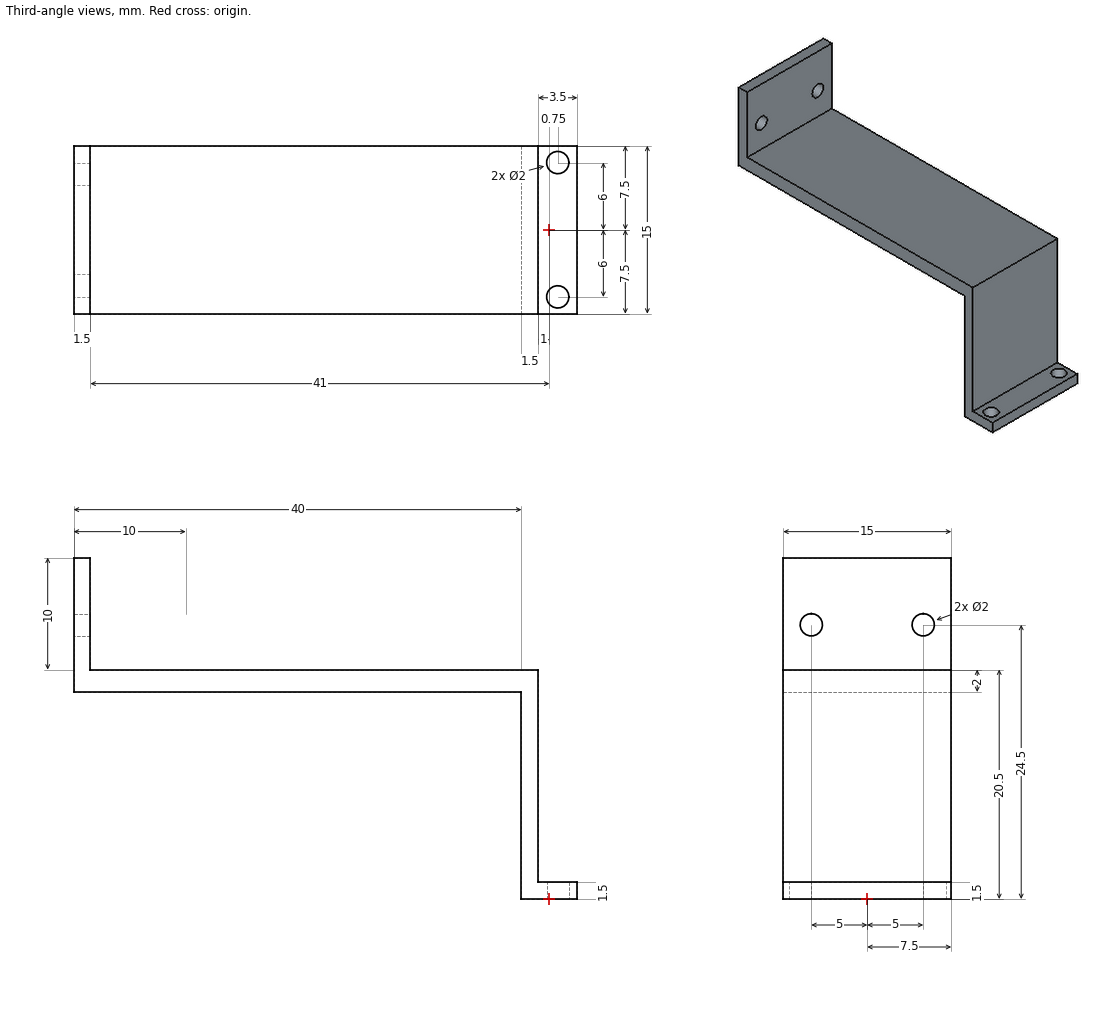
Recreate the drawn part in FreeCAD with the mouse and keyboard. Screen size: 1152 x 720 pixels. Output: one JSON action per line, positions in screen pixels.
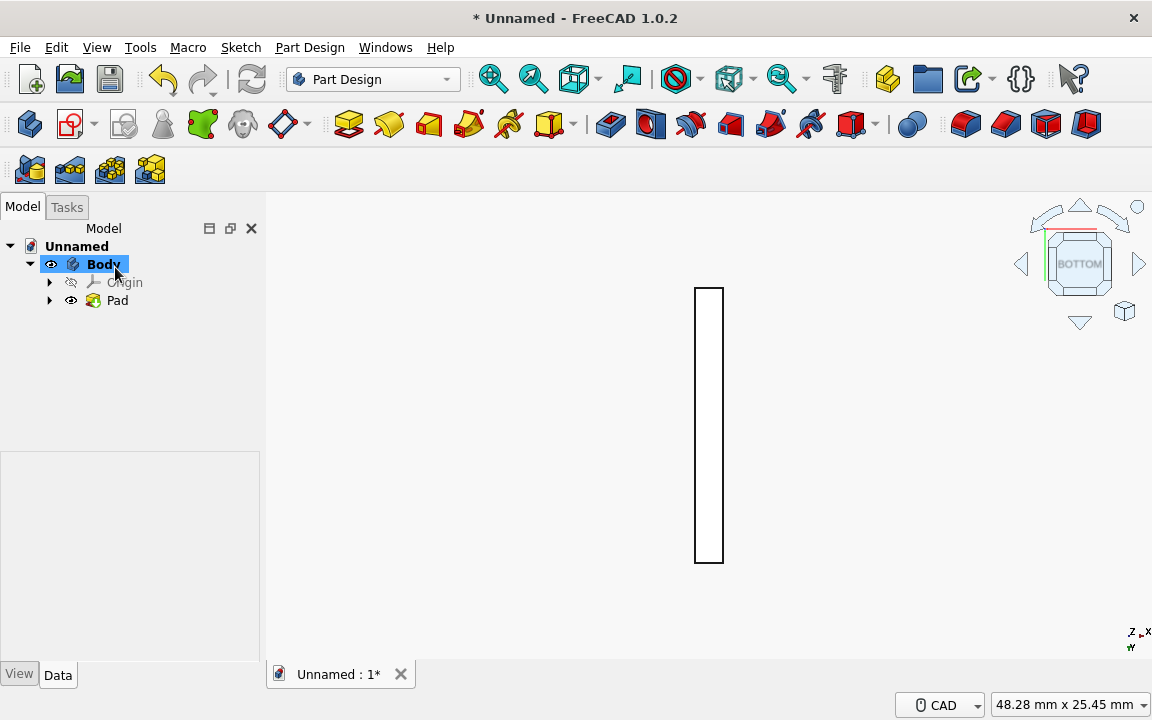
{"action": "left_click", "coordinate": [709, 542]}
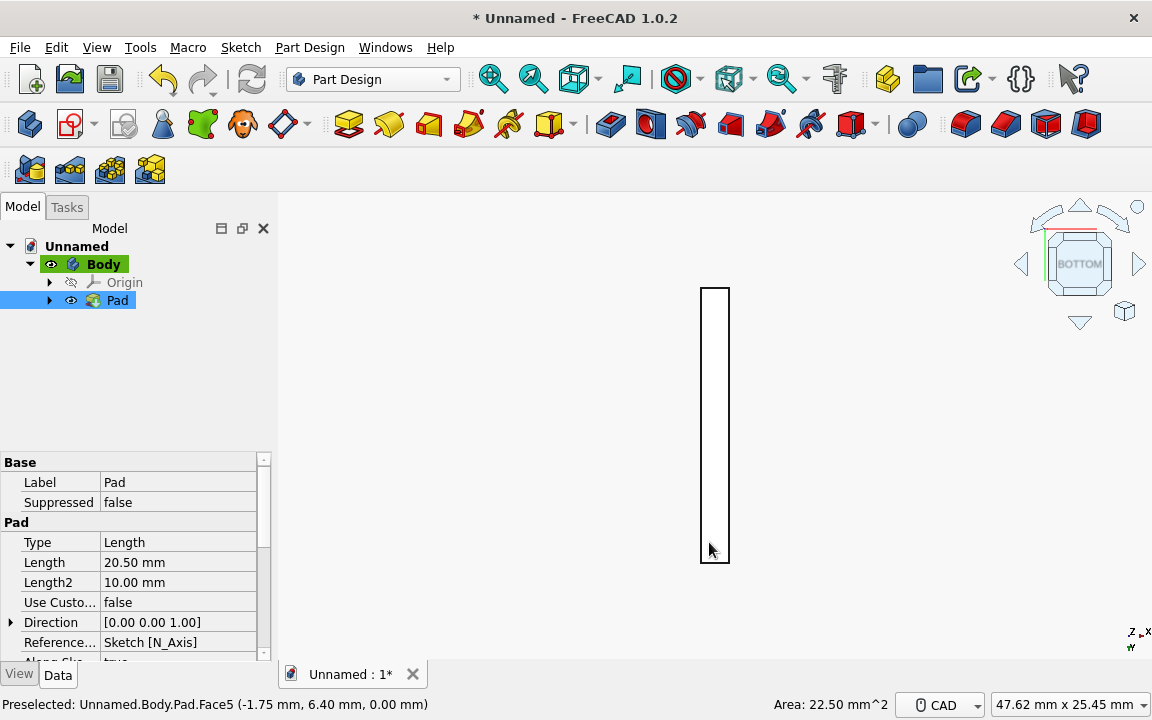
{"action": "left_click", "coordinate": [70, 124]}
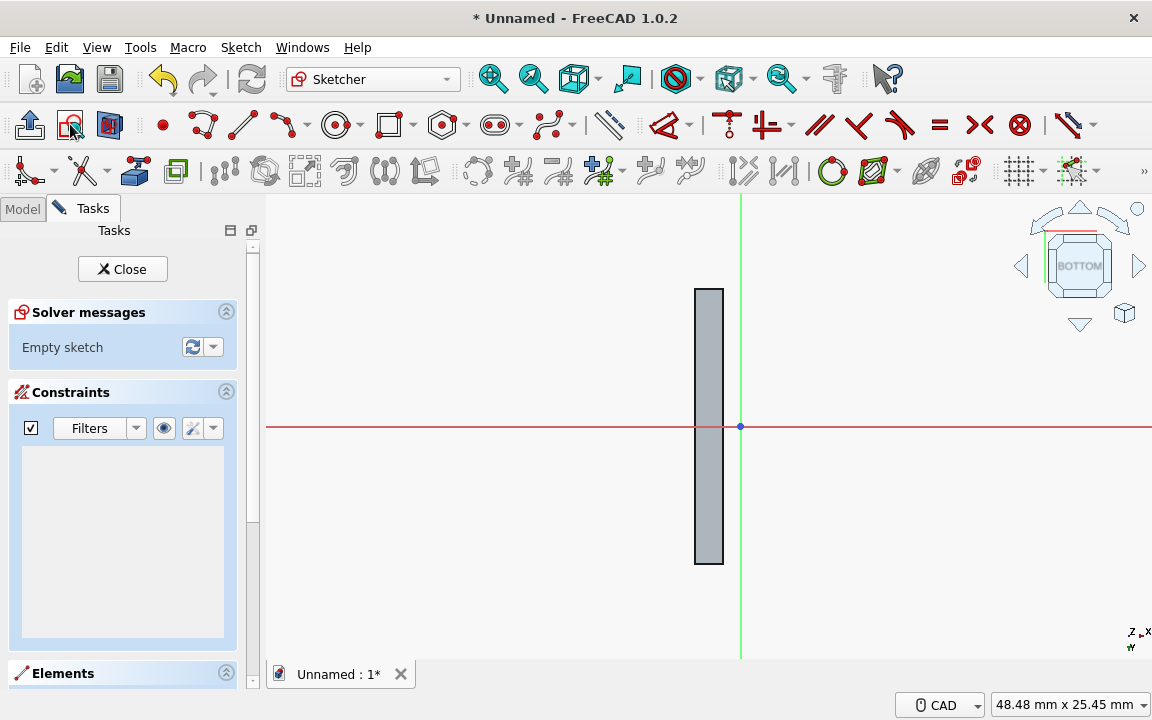
{"action": "left_click", "coordinate": [390, 126]}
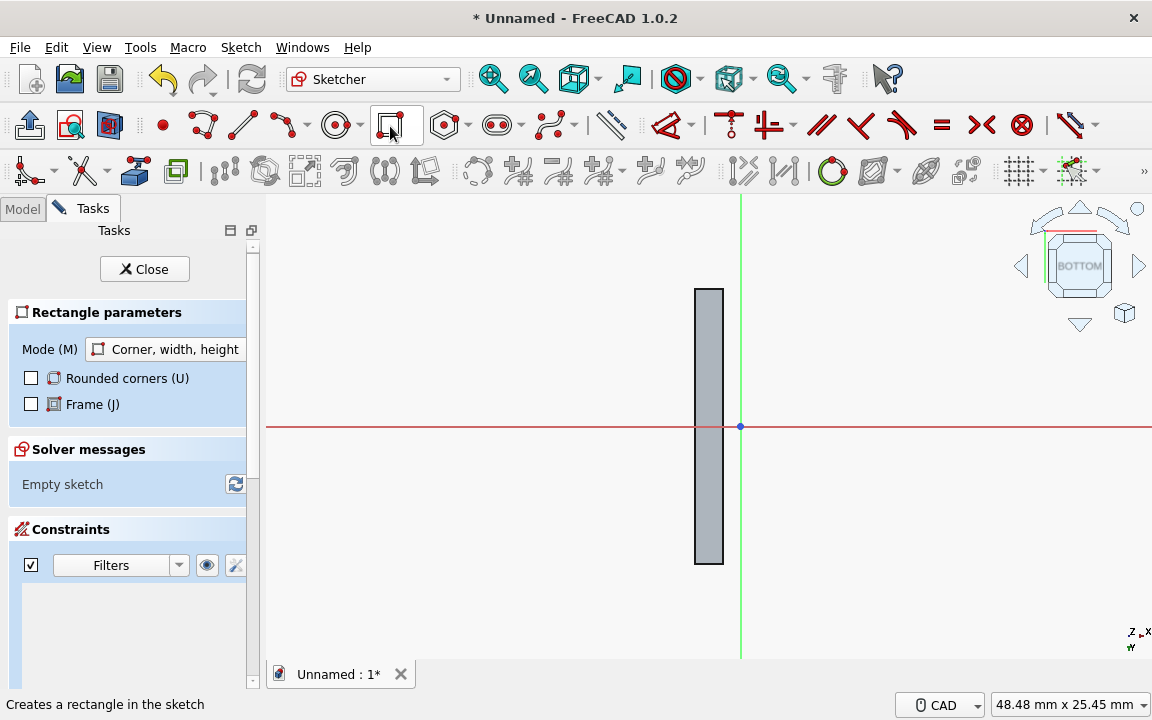
{"action": "left_click", "coordinate": [723, 289]}
{"action": "left_click", "coordinate": [787, 564]}
{"action": "key", "text": "Escape"}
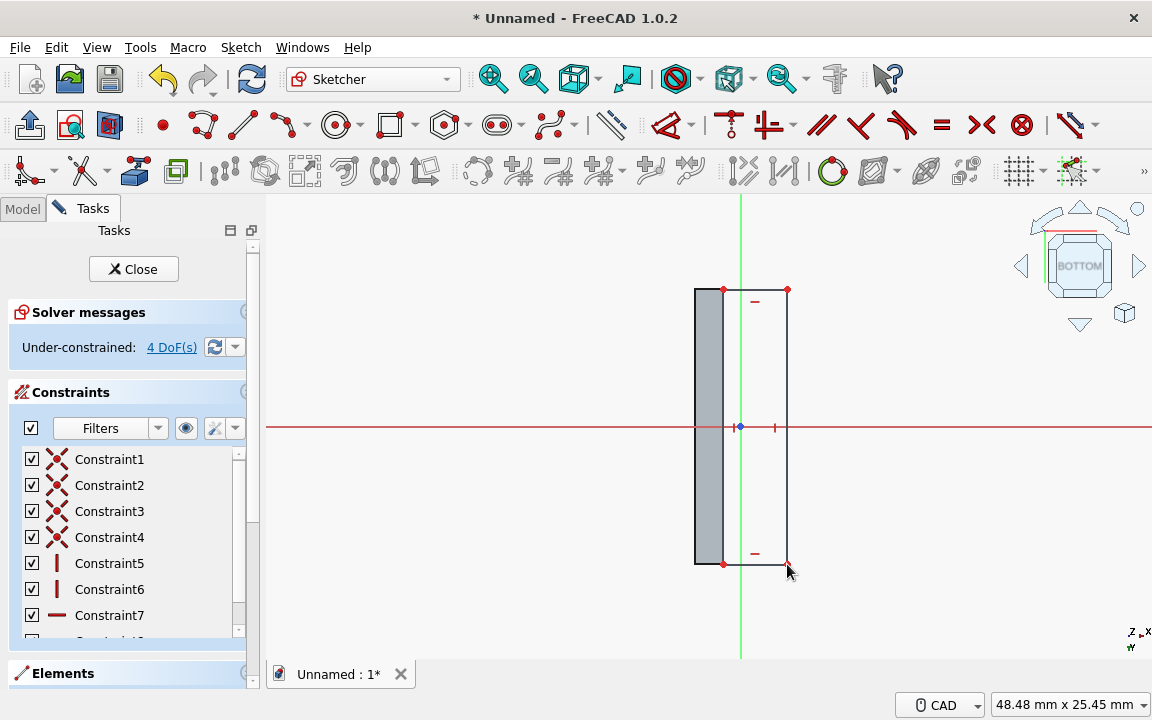
{"action": "left_click", "coordinate": [666, 126]}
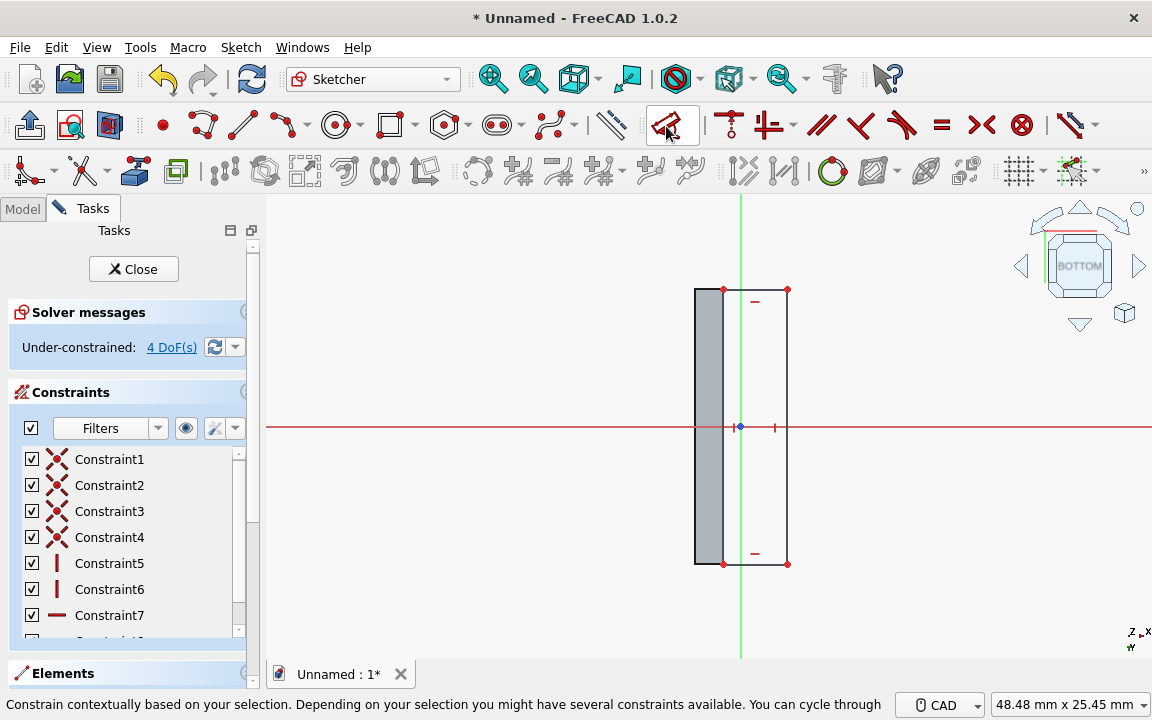
{"action": "left_click", "coordinate": [723, 372]}
{"action": "left_click", "coordinate": [689, 364]}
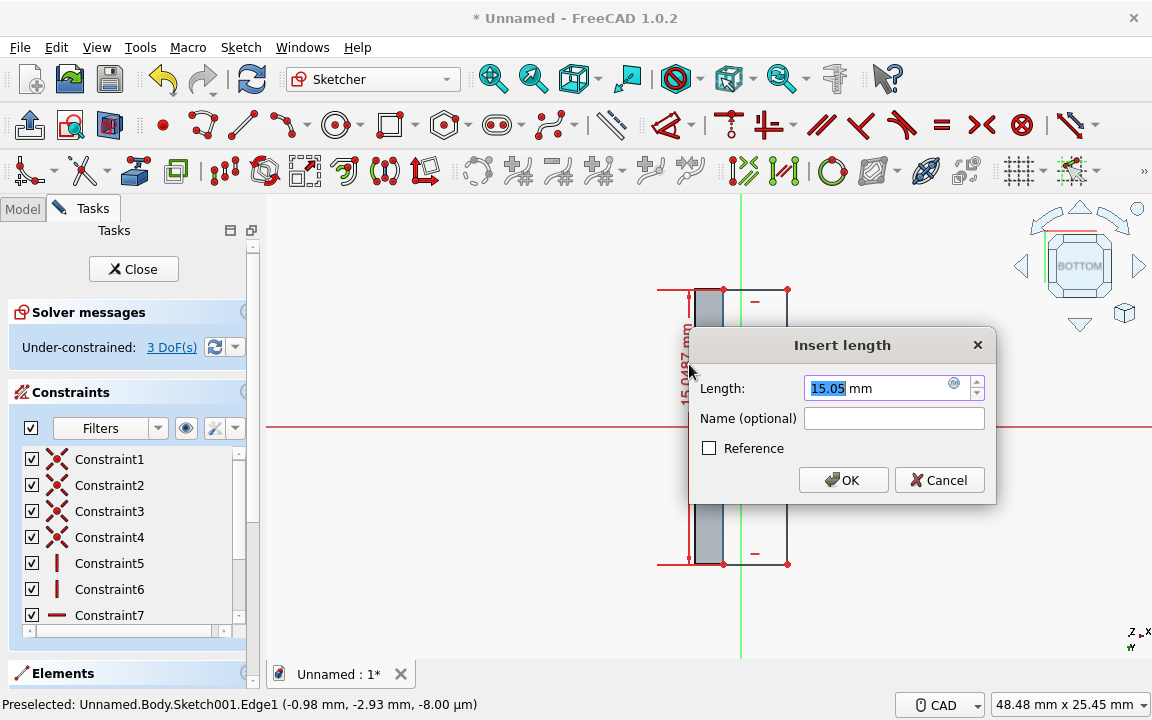
{"action": "type", "text": "15"}
{"action": "key", "text": "Return"}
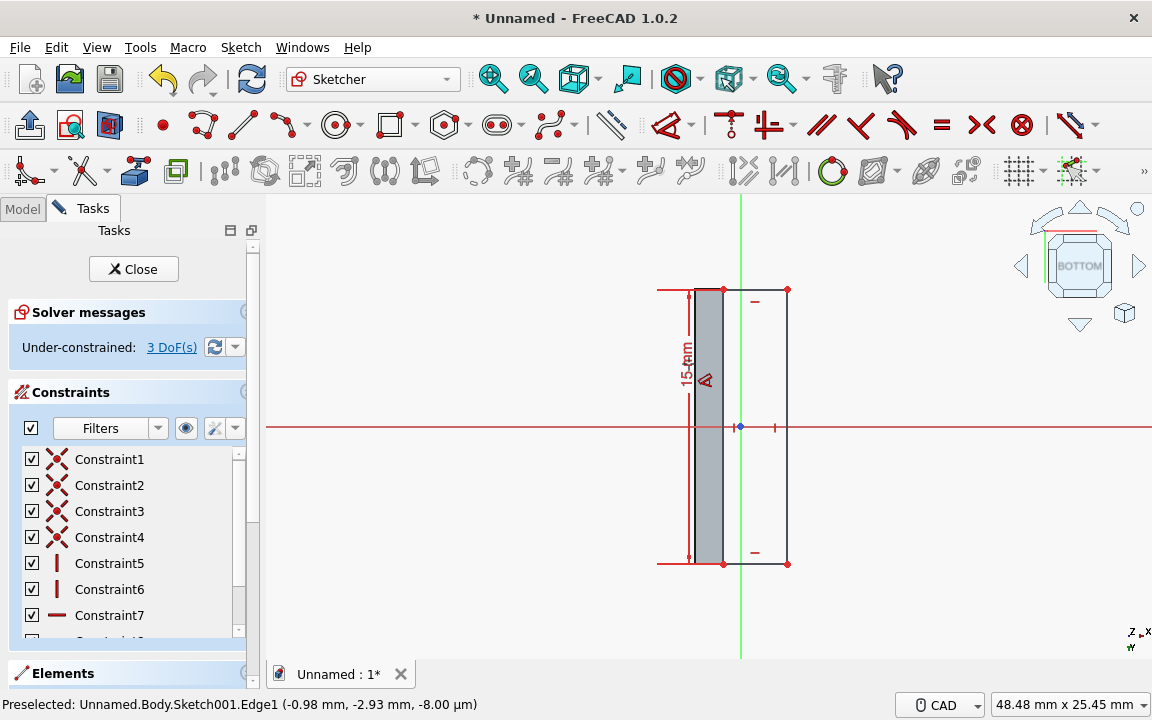
{"action": "scroll", "coordinate": [723, 290], "scroll_direction": "up", "scroll_amount": 4}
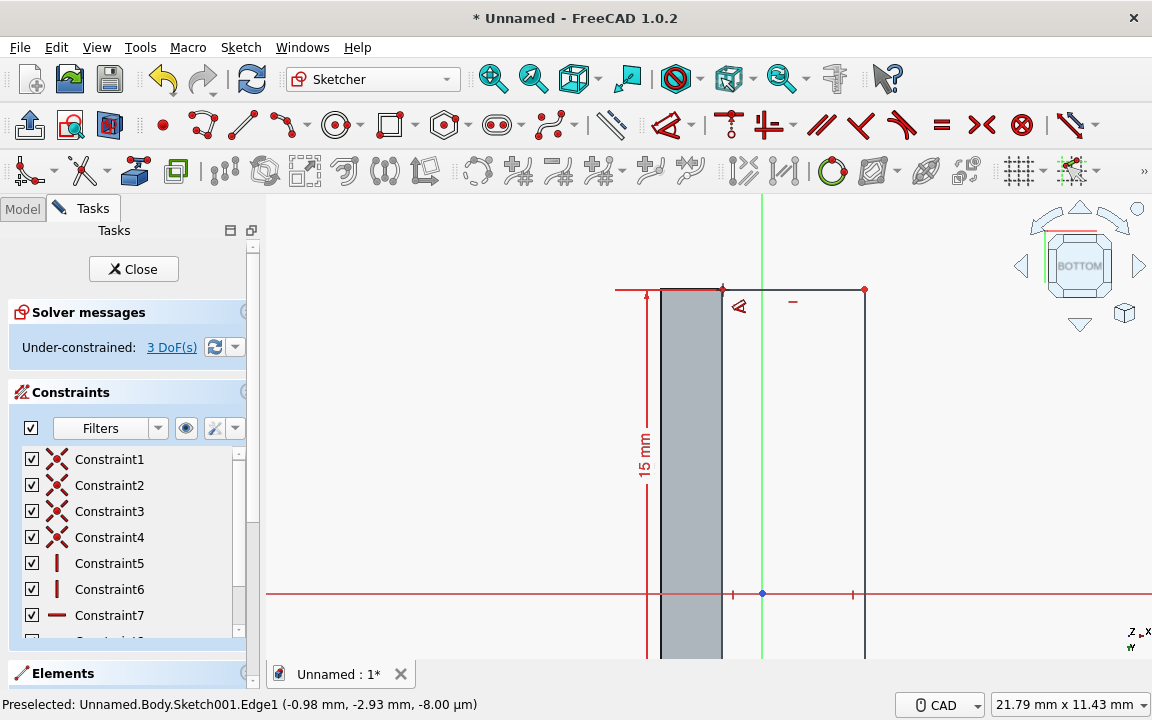
{"action": "left_click", "coordinate": [722, 290]}
{"action": "left_click", "coordinate": [742, 256]}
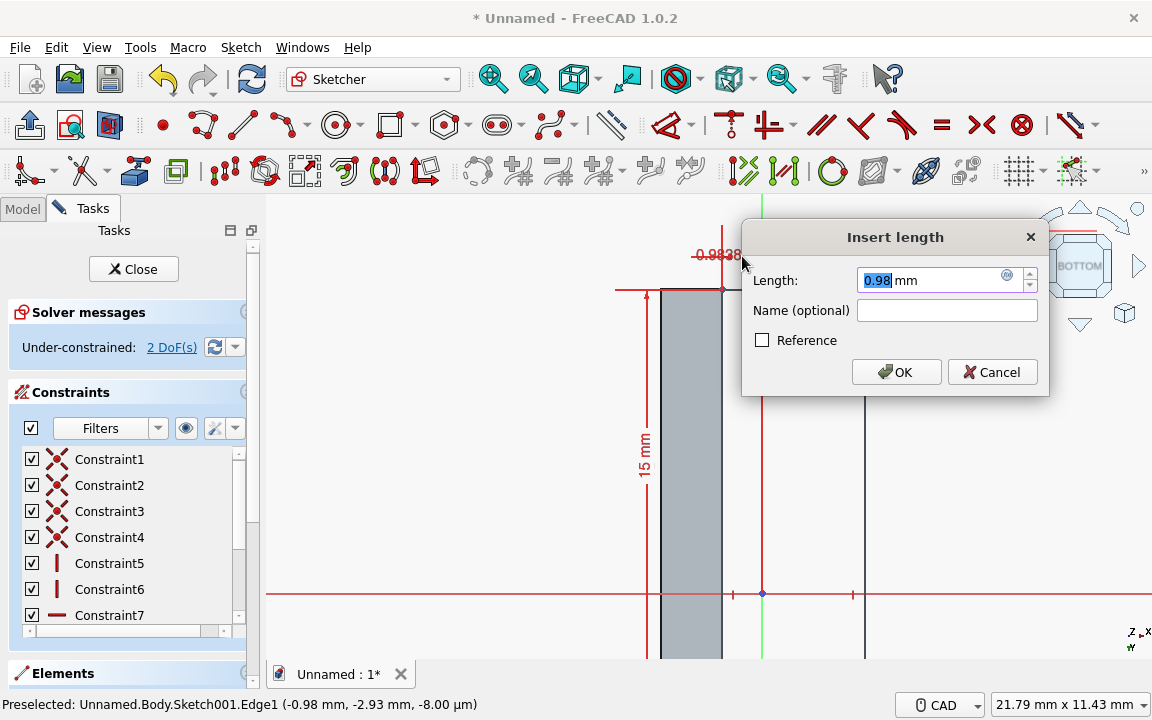
{"action": "type", "text": "1"}
{"action": "key", "text": "Return"}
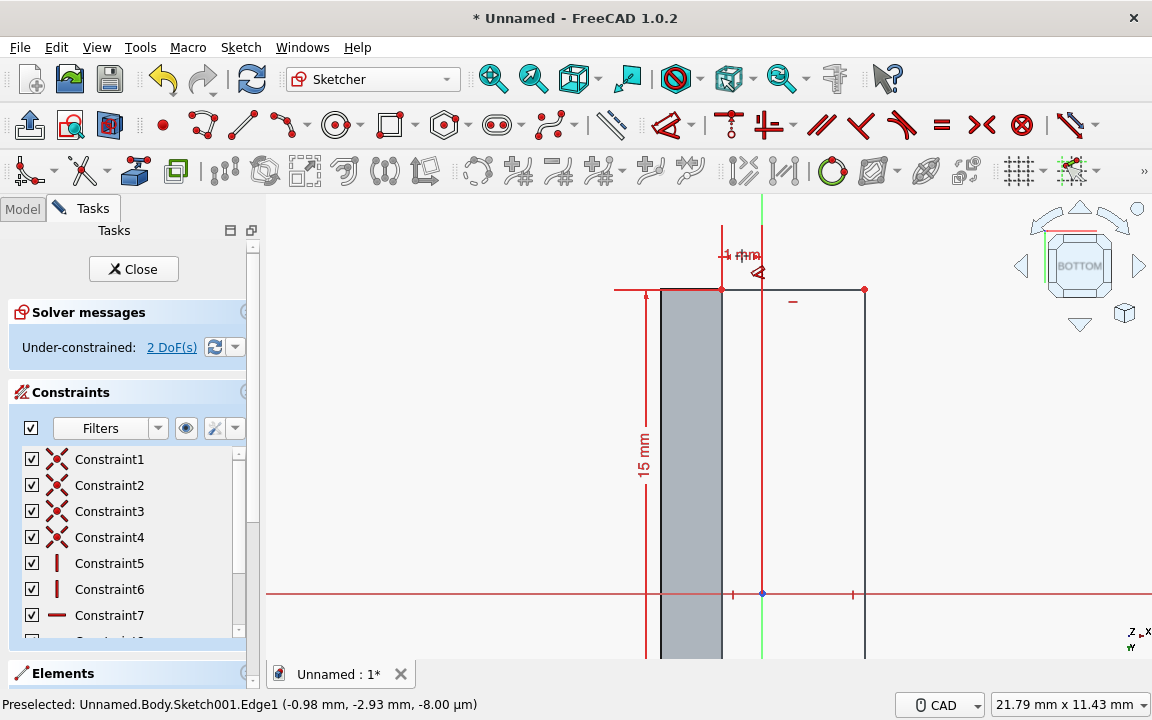
{"action": "scroll", "coordinate": [516, 290], "scroll_direction": "down", "scroll_amount": 4}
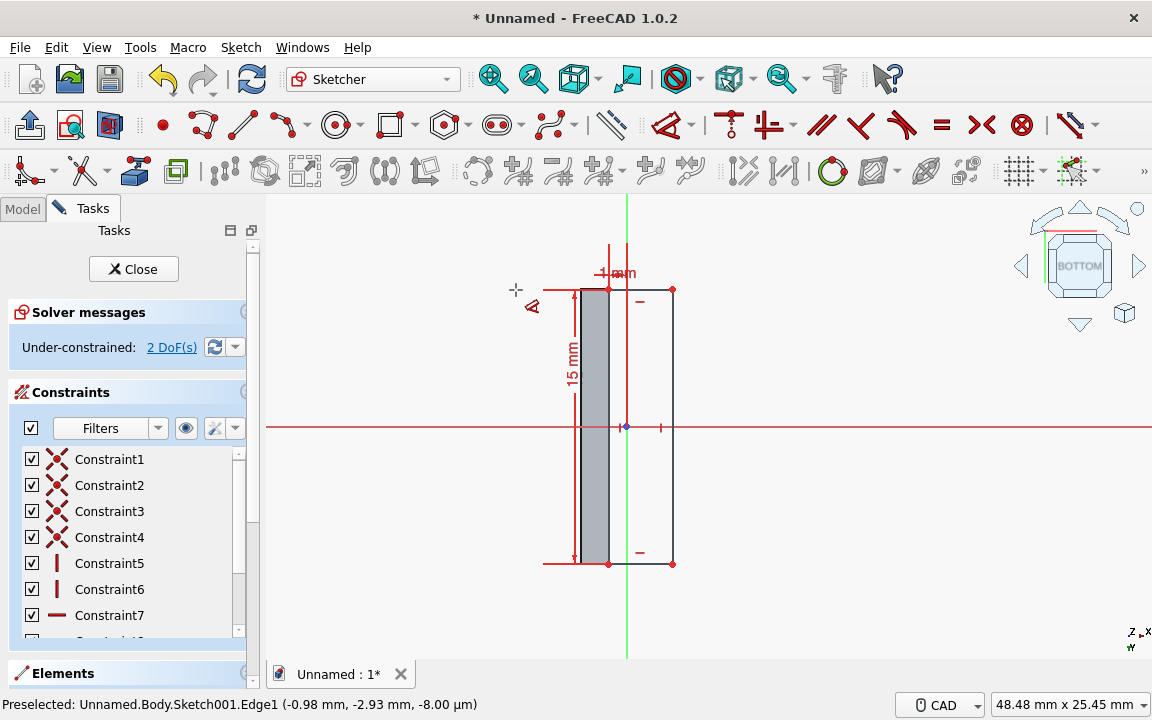
{"action": "left_click", "coordinate": [628, 564]}
{"action": "left_click", "coordinate": [641, 598]}